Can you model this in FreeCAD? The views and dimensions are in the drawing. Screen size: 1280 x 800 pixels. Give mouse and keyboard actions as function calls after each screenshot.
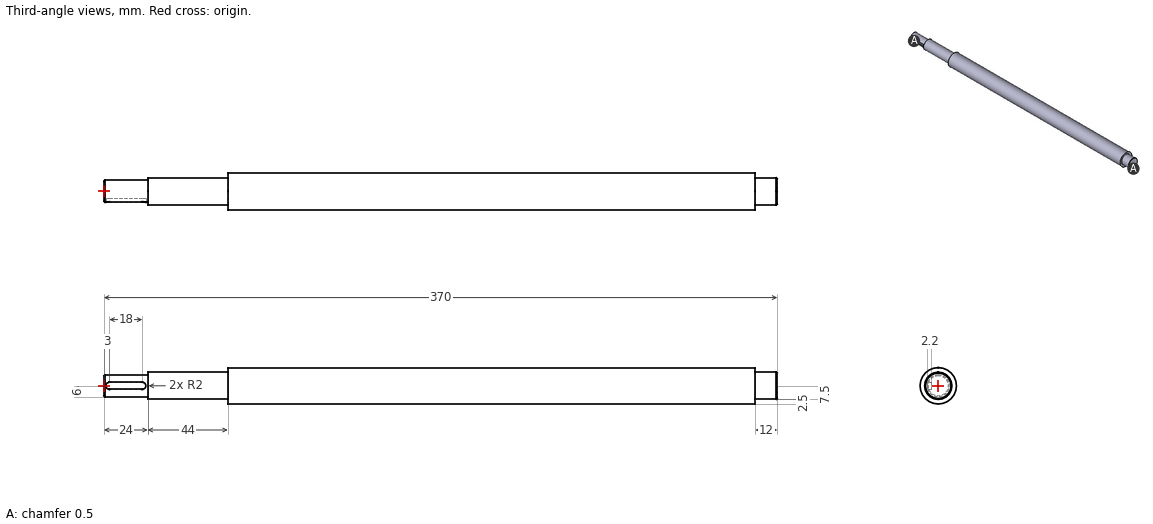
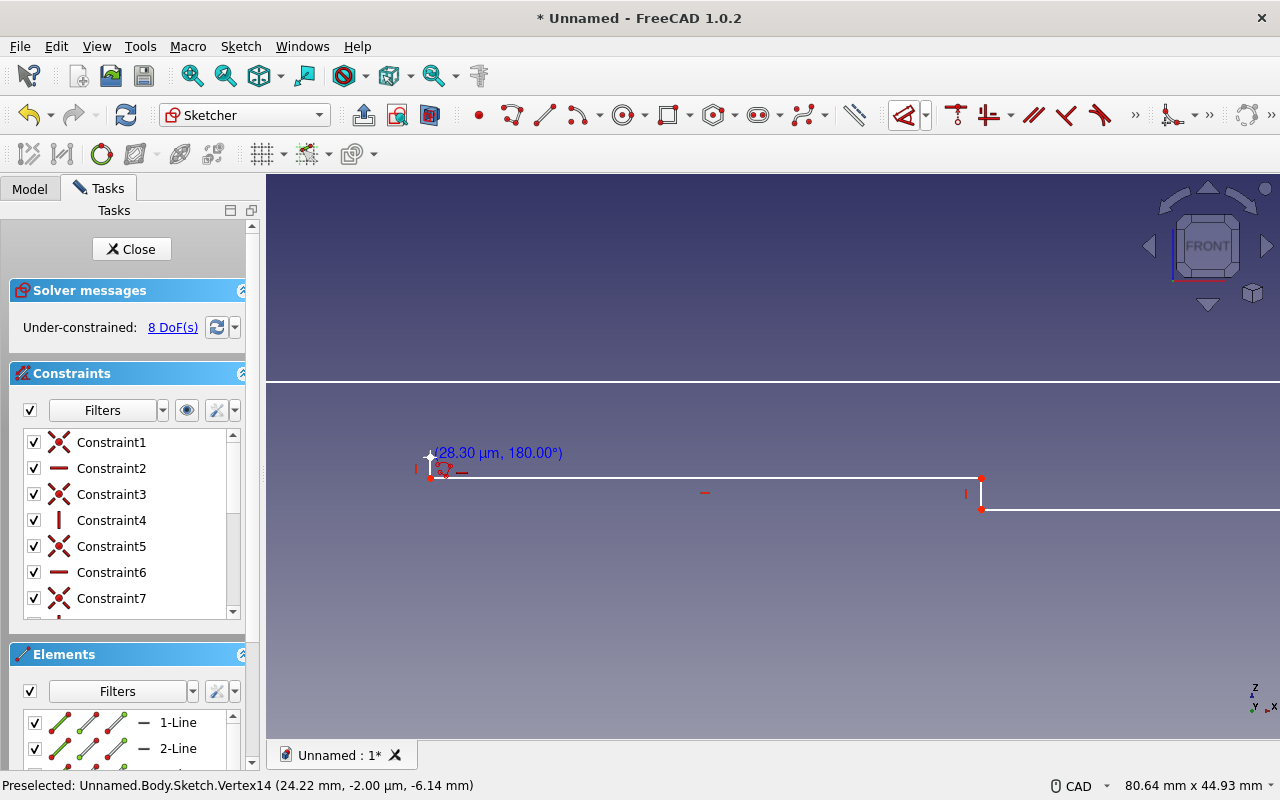
scroll(431, 458, down, 10)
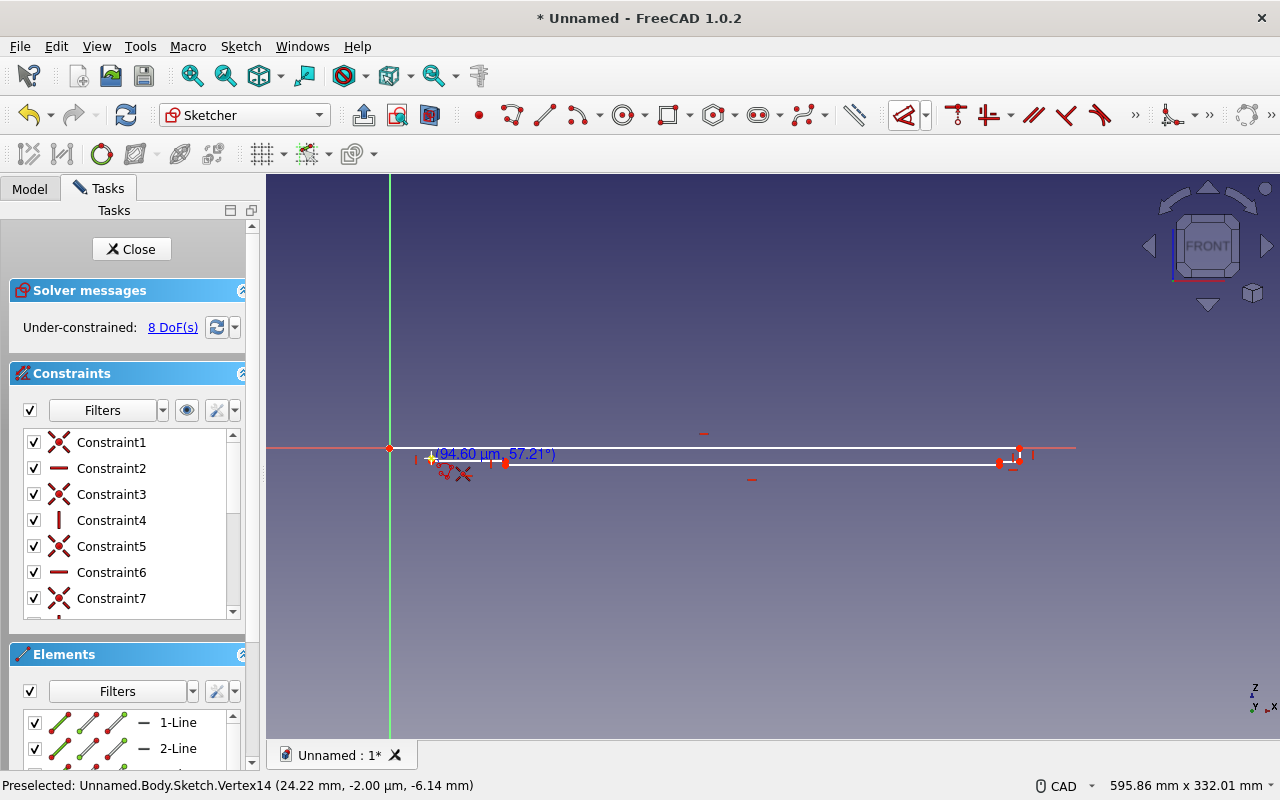
scroll(390, 458, up, 3)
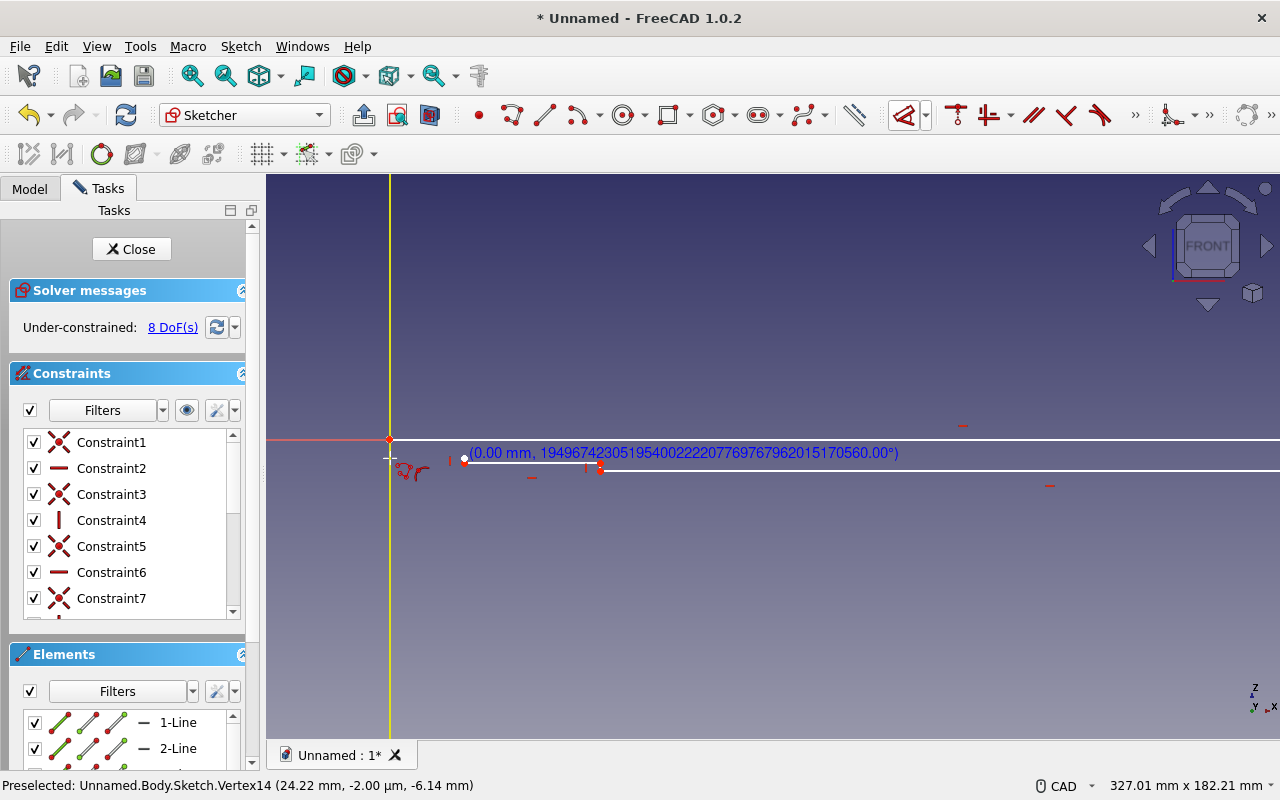
click(399, 458)
click(390, 440)
key(Escape)
key(Escape)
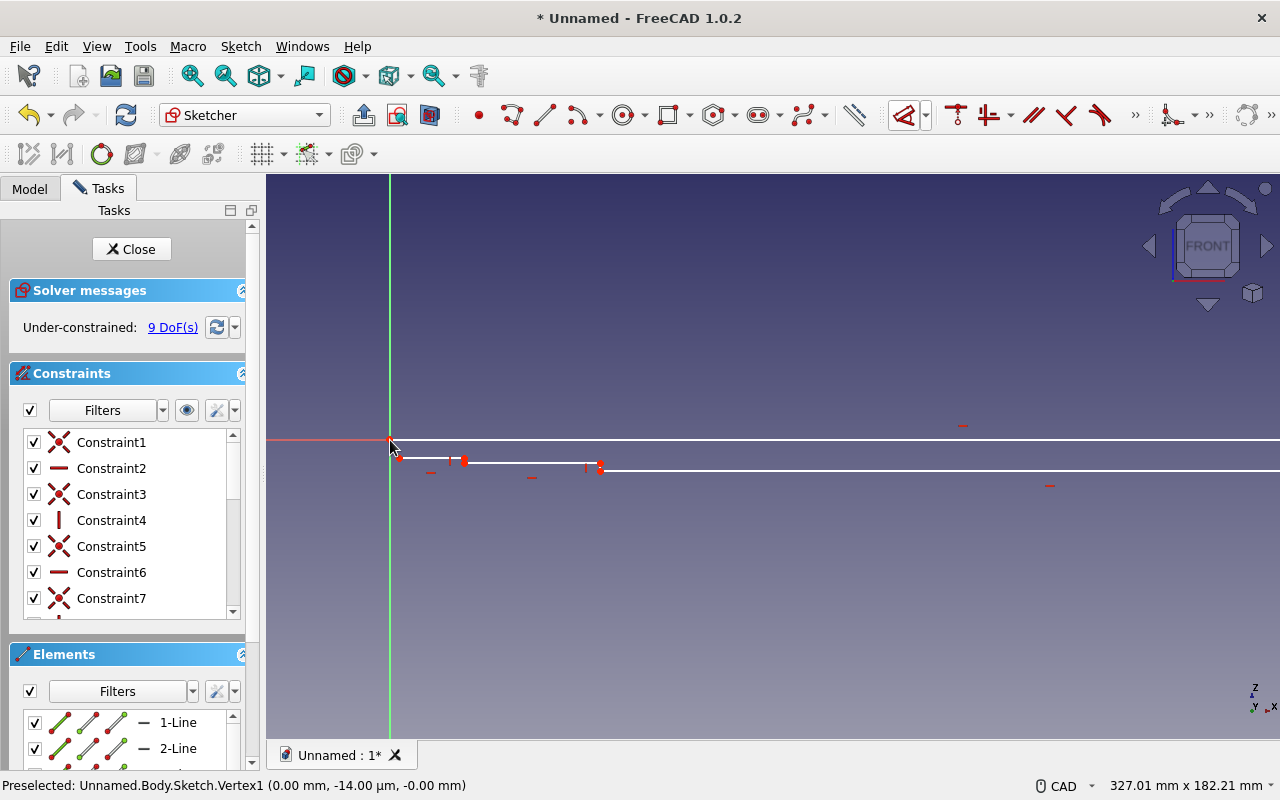
scroll(393, 447, up, 4)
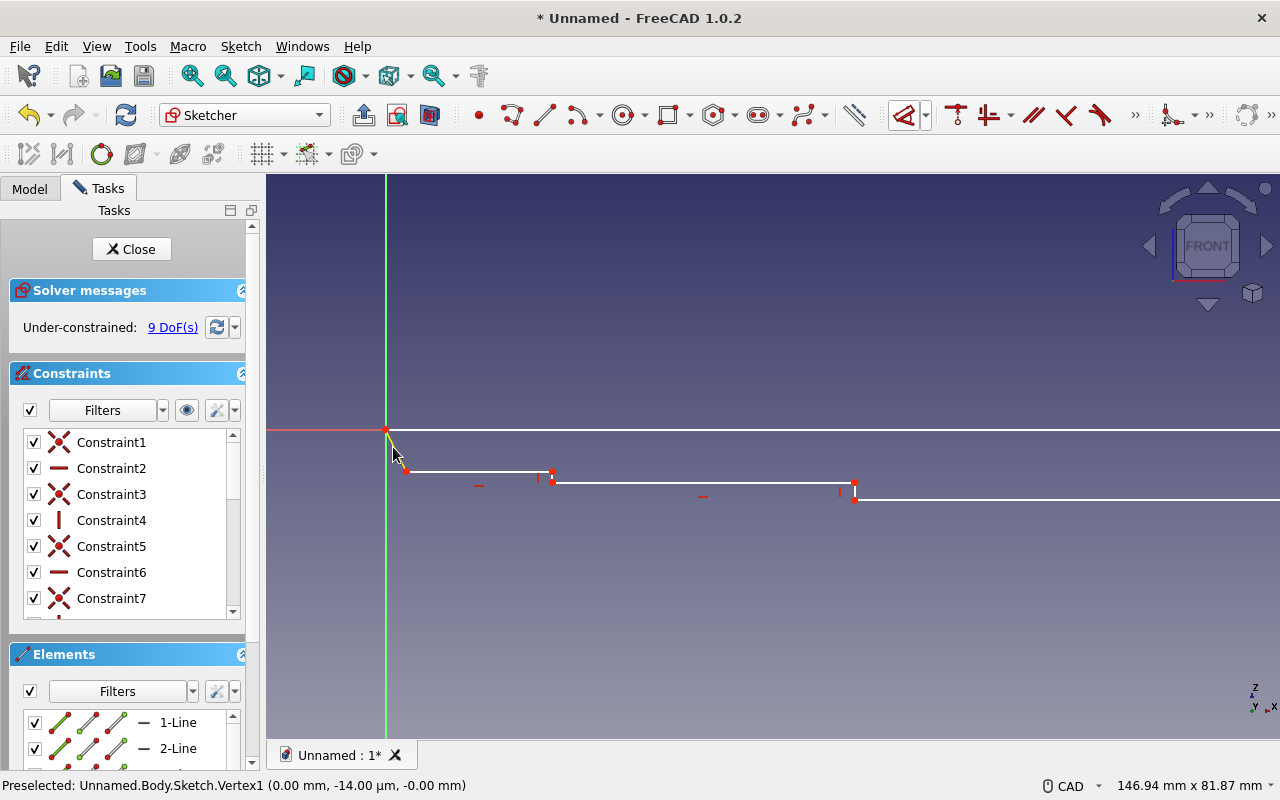
click(394, 447)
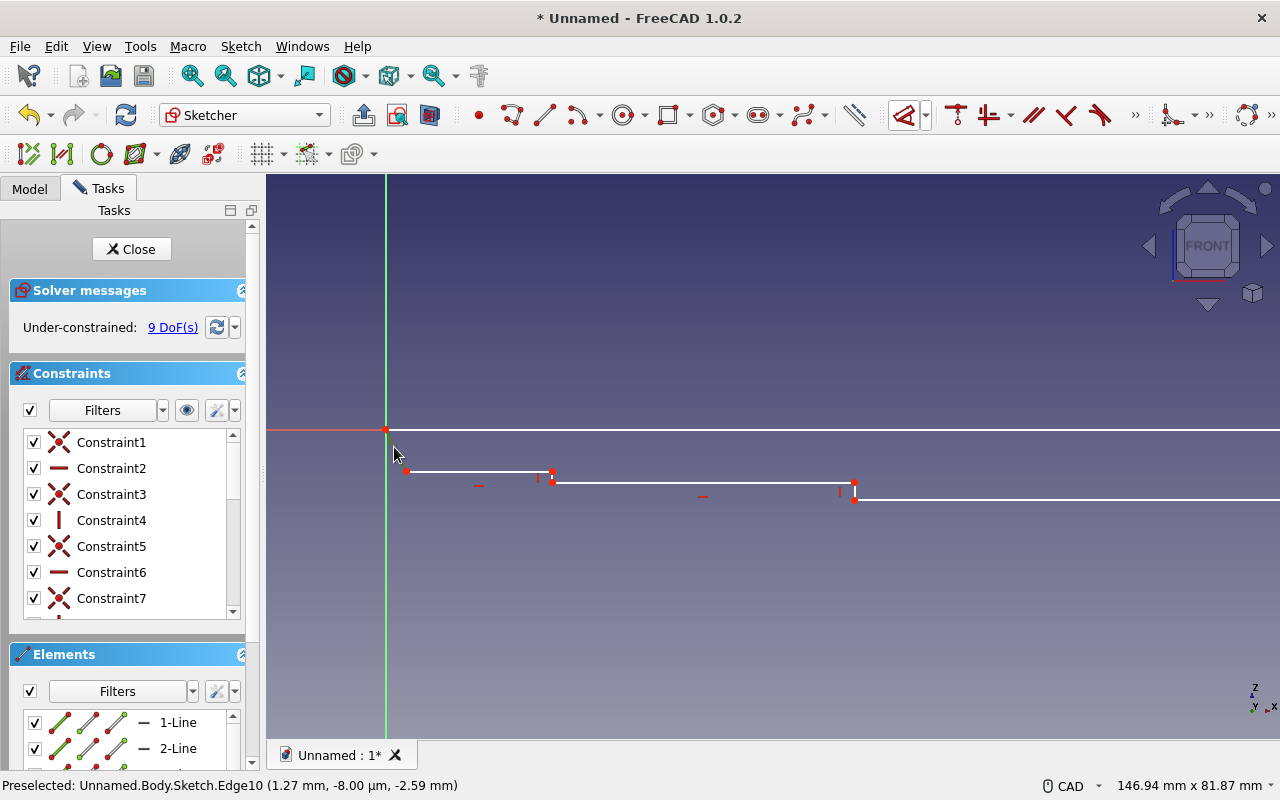
key(v)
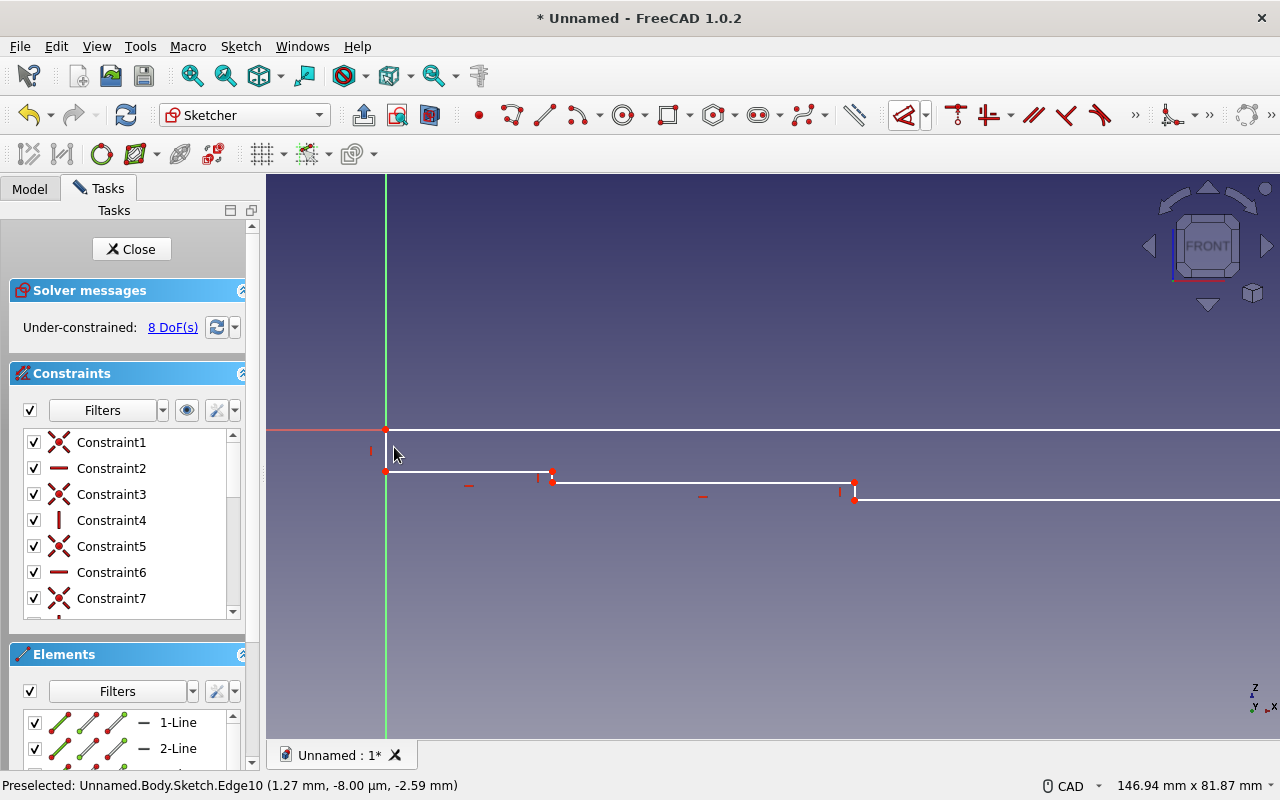
key(d)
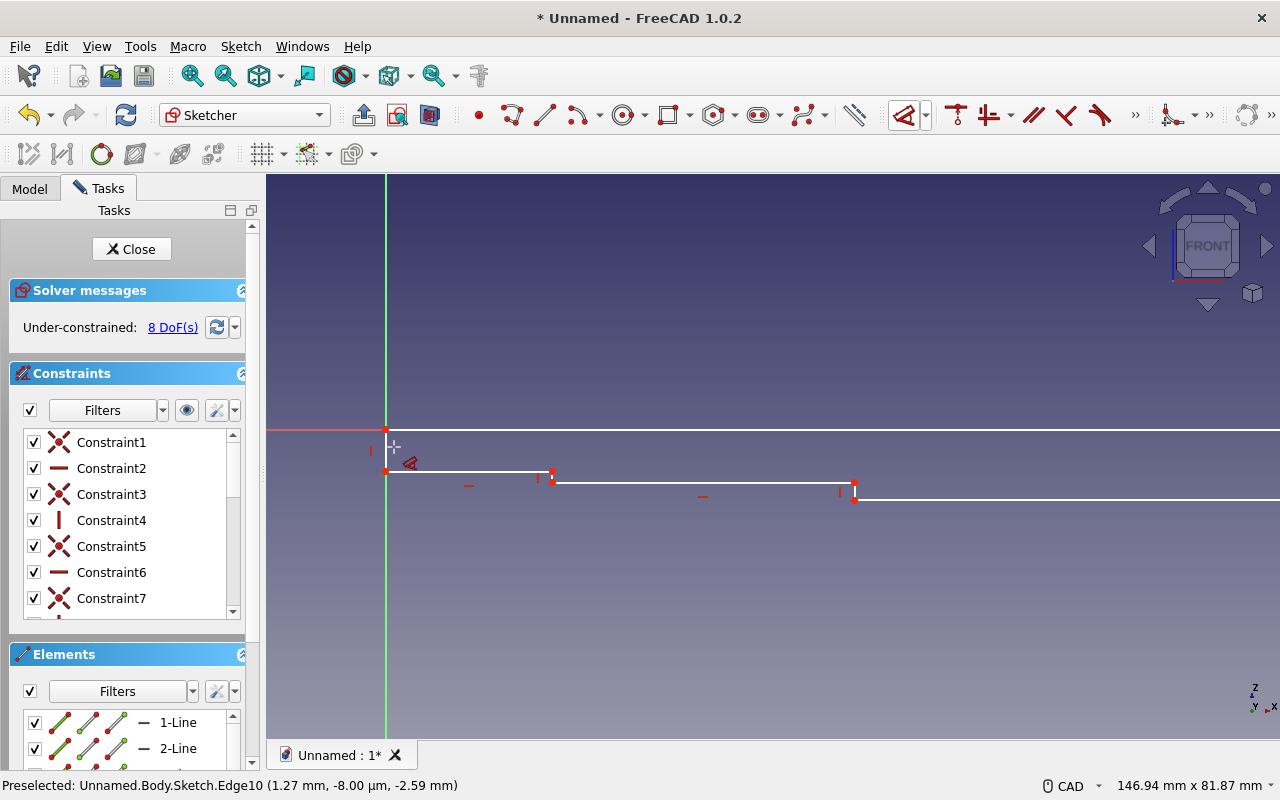
click(386, 459)
click(352, 451)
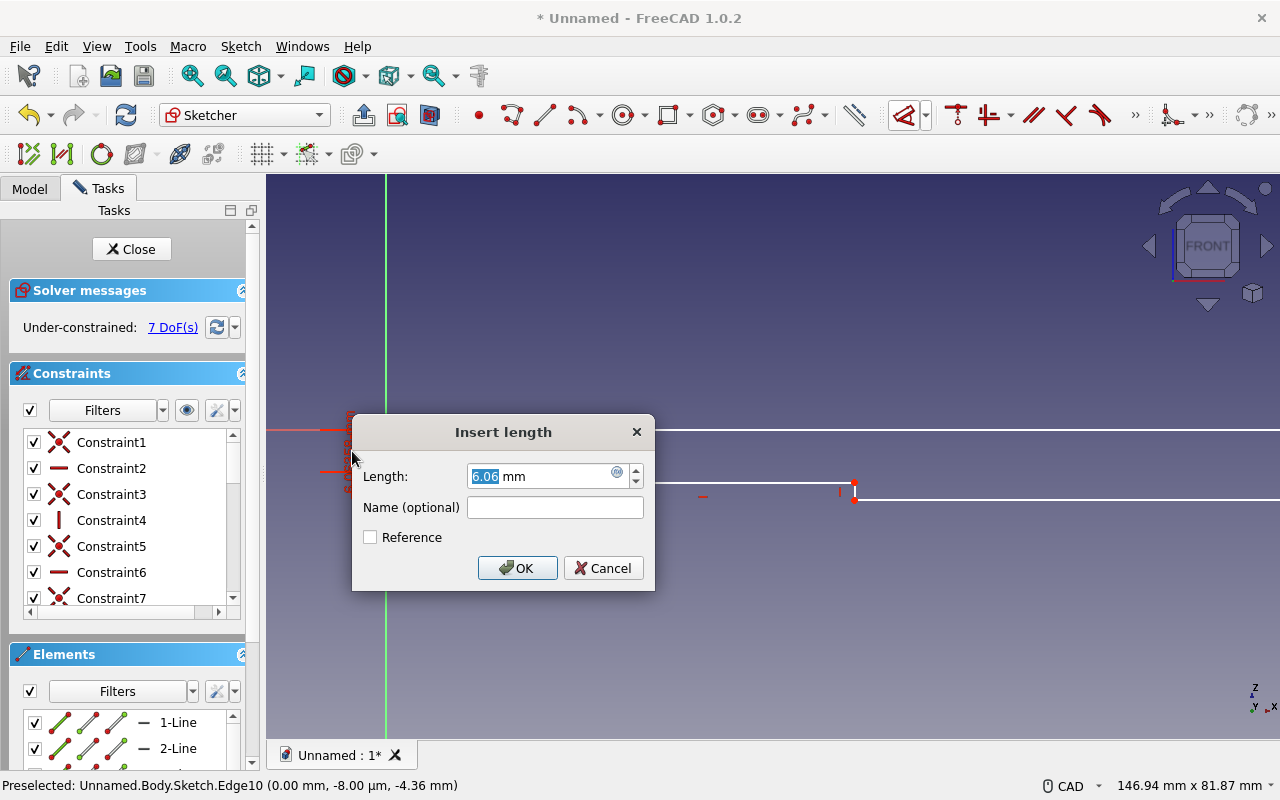
text(6)
key(Return)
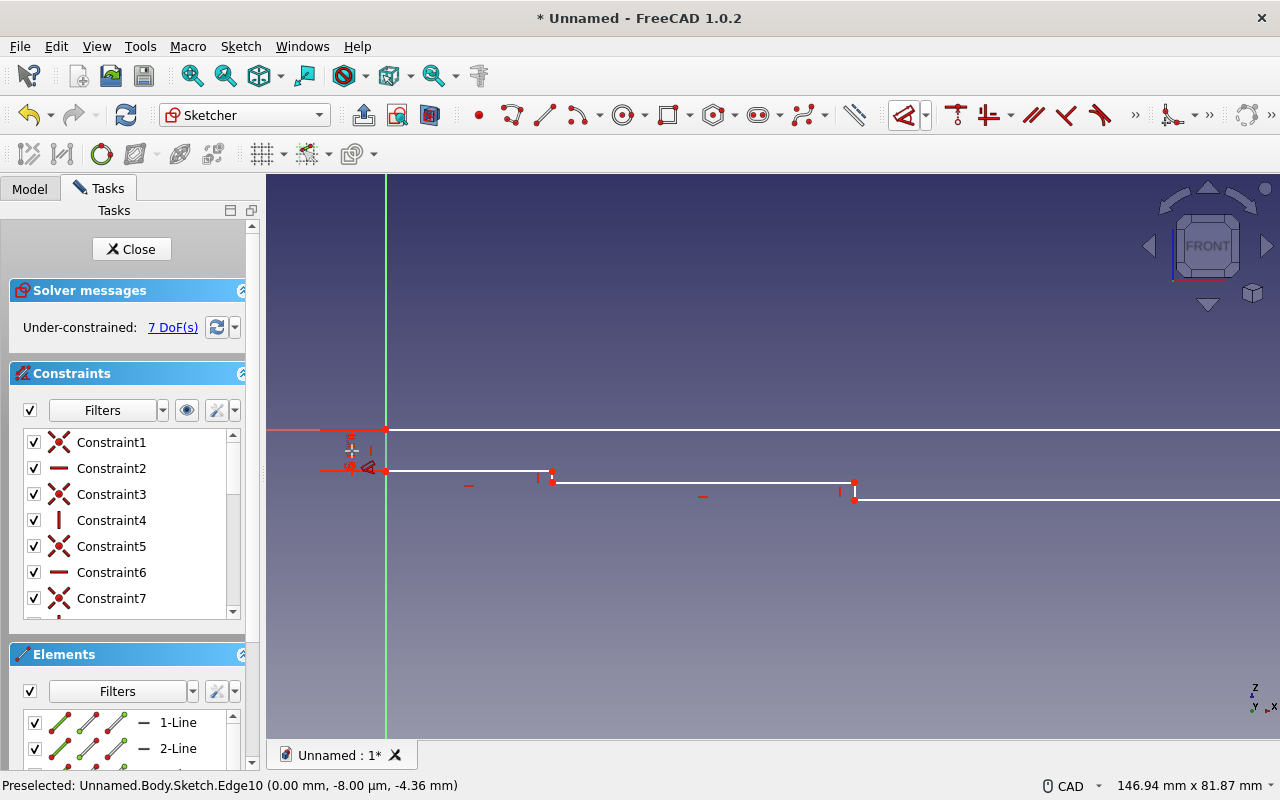
scroll(391, 454, down, 7)